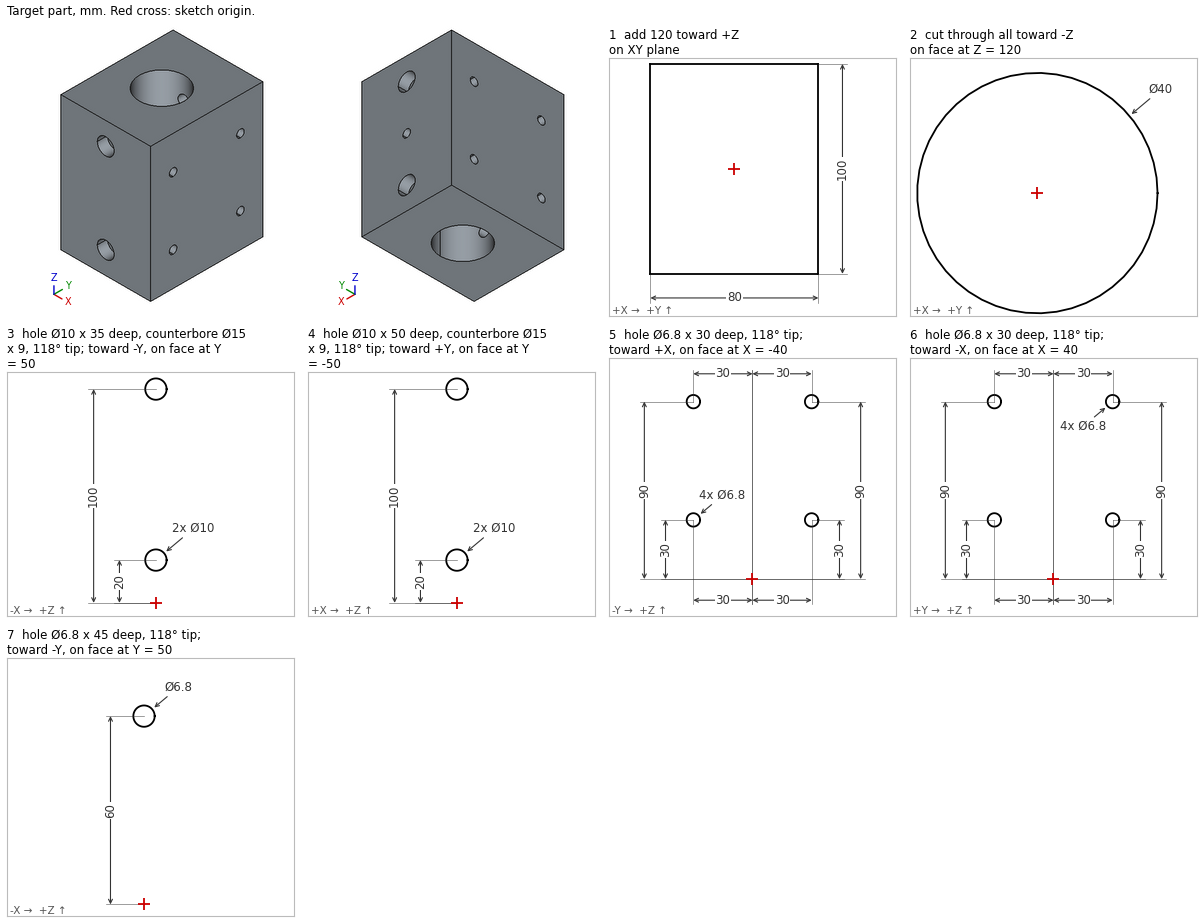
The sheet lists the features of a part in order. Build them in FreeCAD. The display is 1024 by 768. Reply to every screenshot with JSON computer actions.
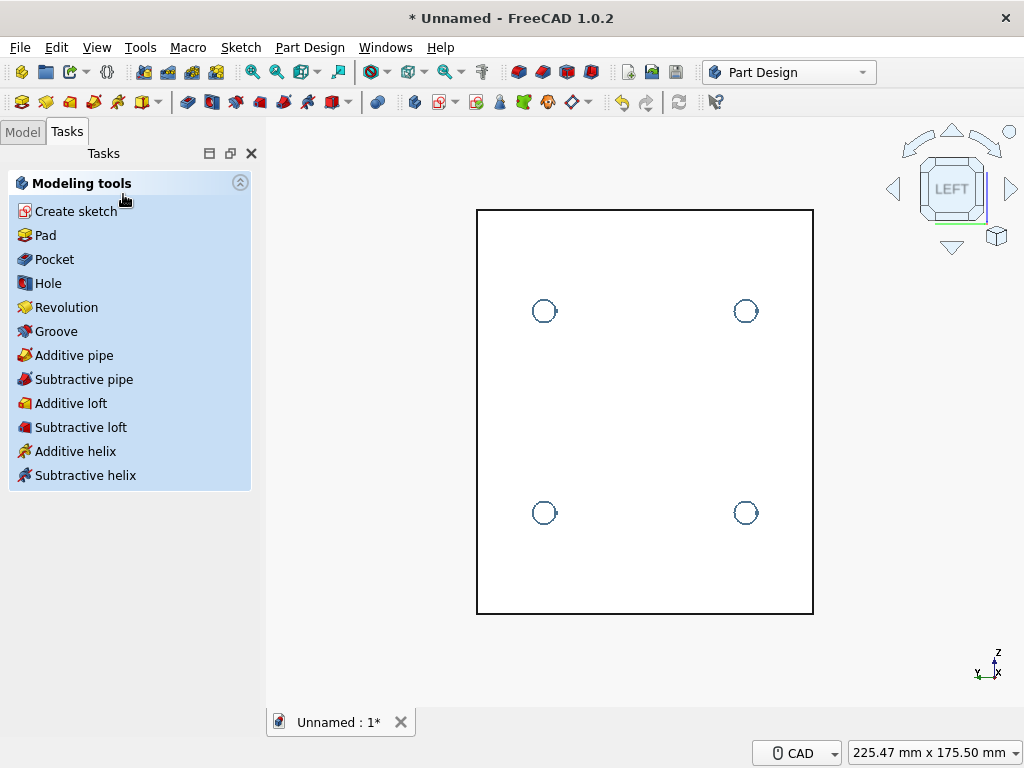
{"action": "left_click", "coordinate": [212, 102]}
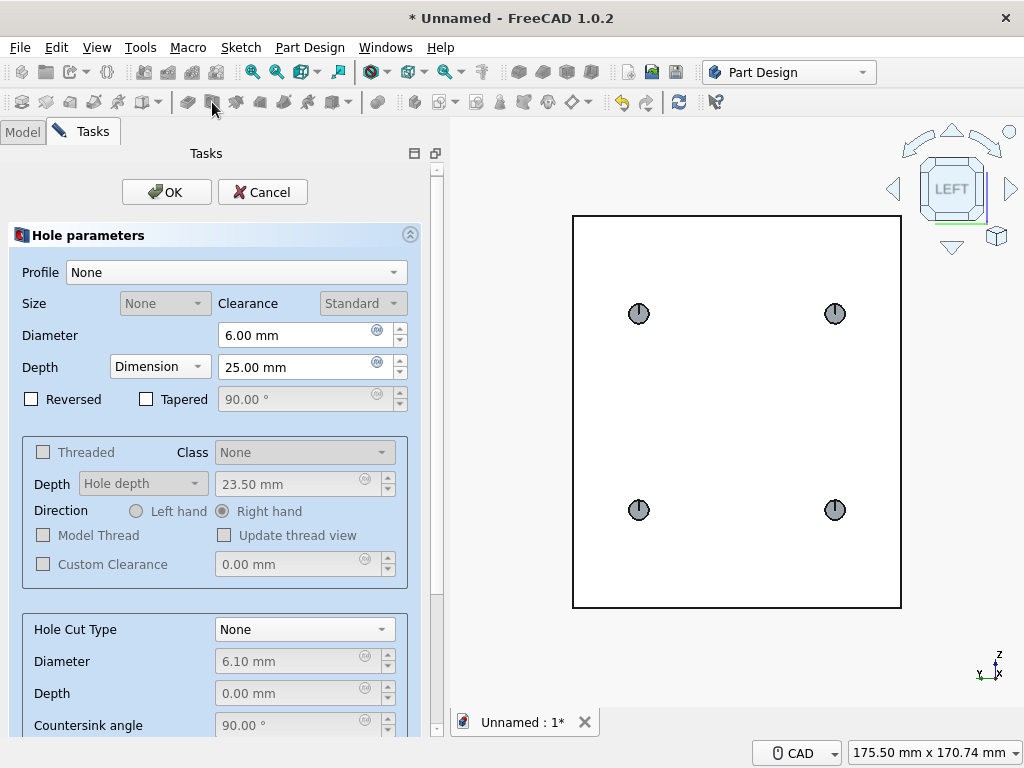
{"action": "triple_click", "coordinate": [305, 335]}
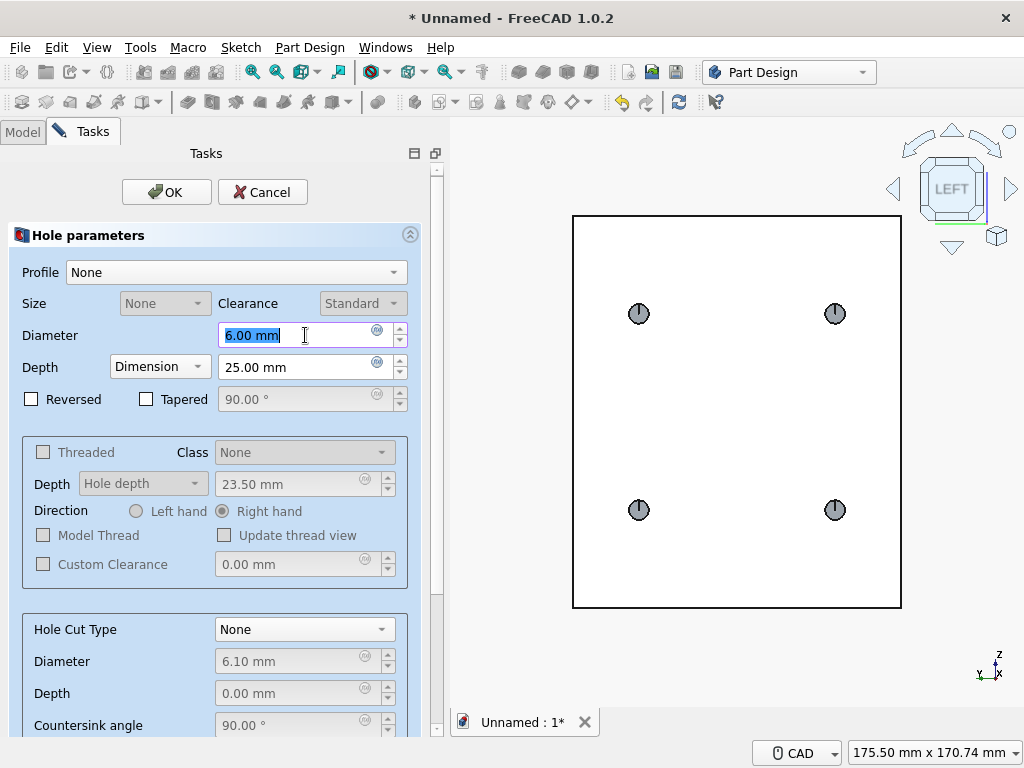
{"action": "type", "text": "6.8"}
{"action": "key", "text": "Tab"}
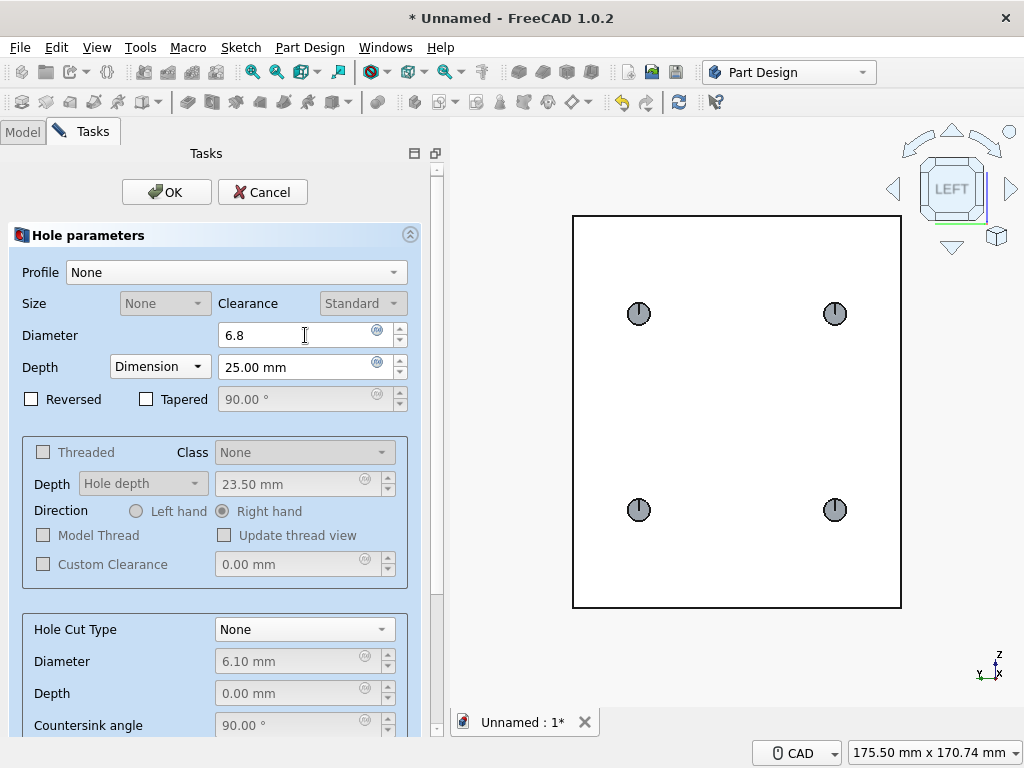
{"action": "triple_click", "coordinate": [305, 367]}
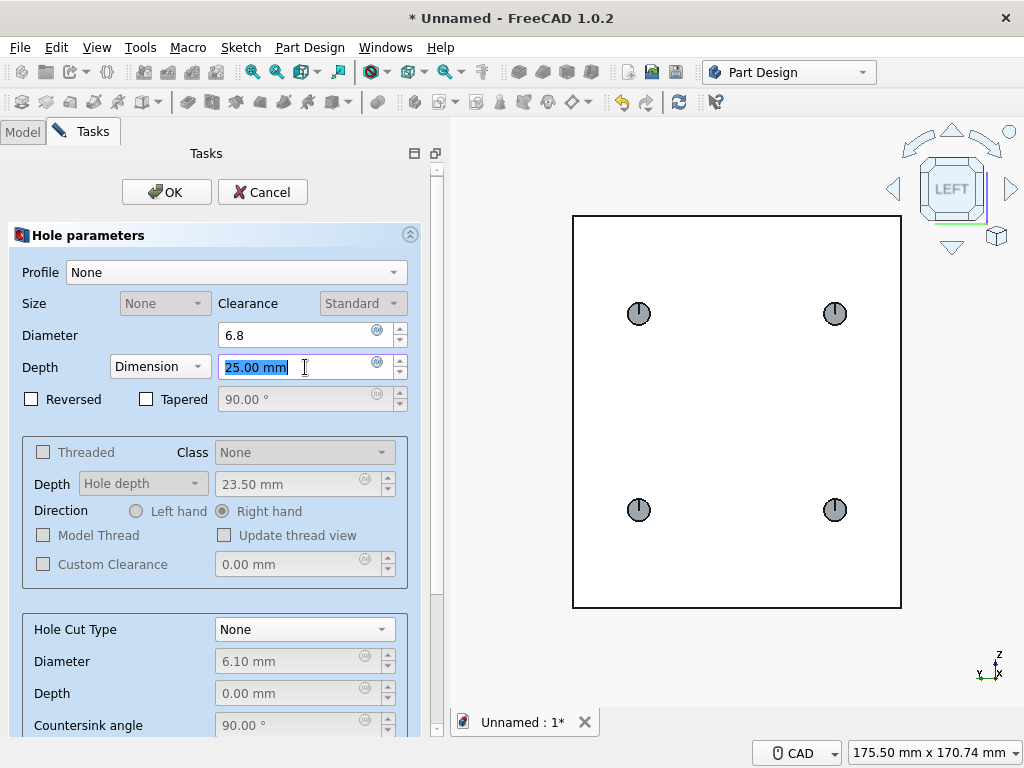
{"action": "type", "text": "30"}
{"action": "key", "text": "Tab"}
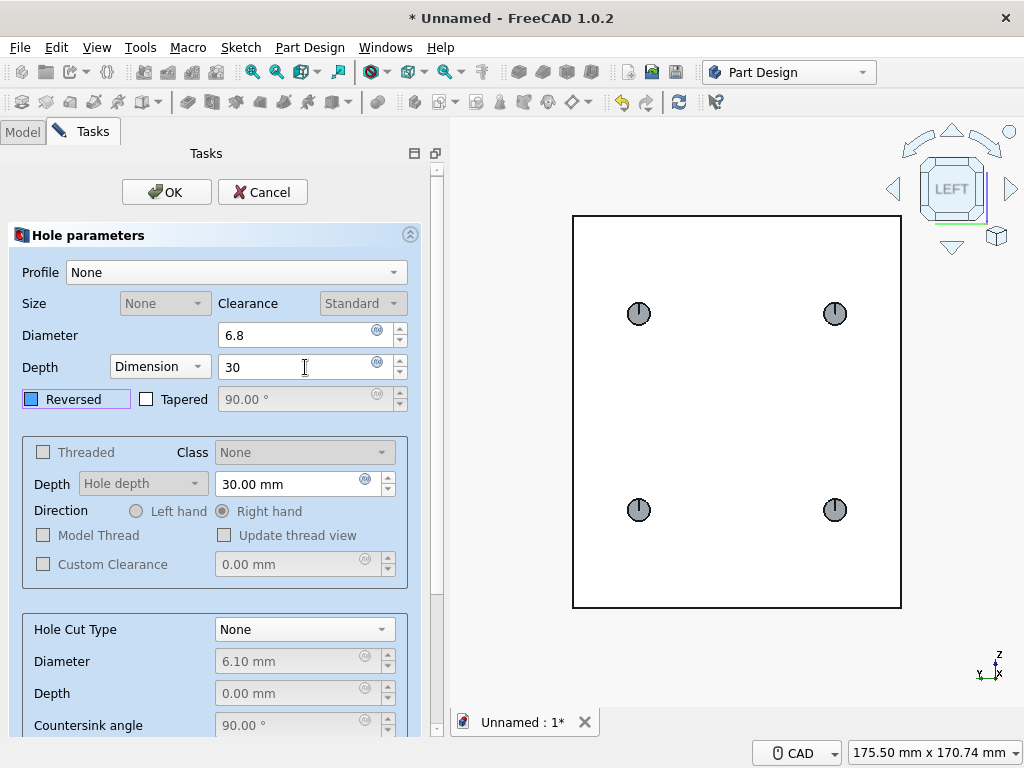
{"action": "left_click", "coordinate": [167, 192]}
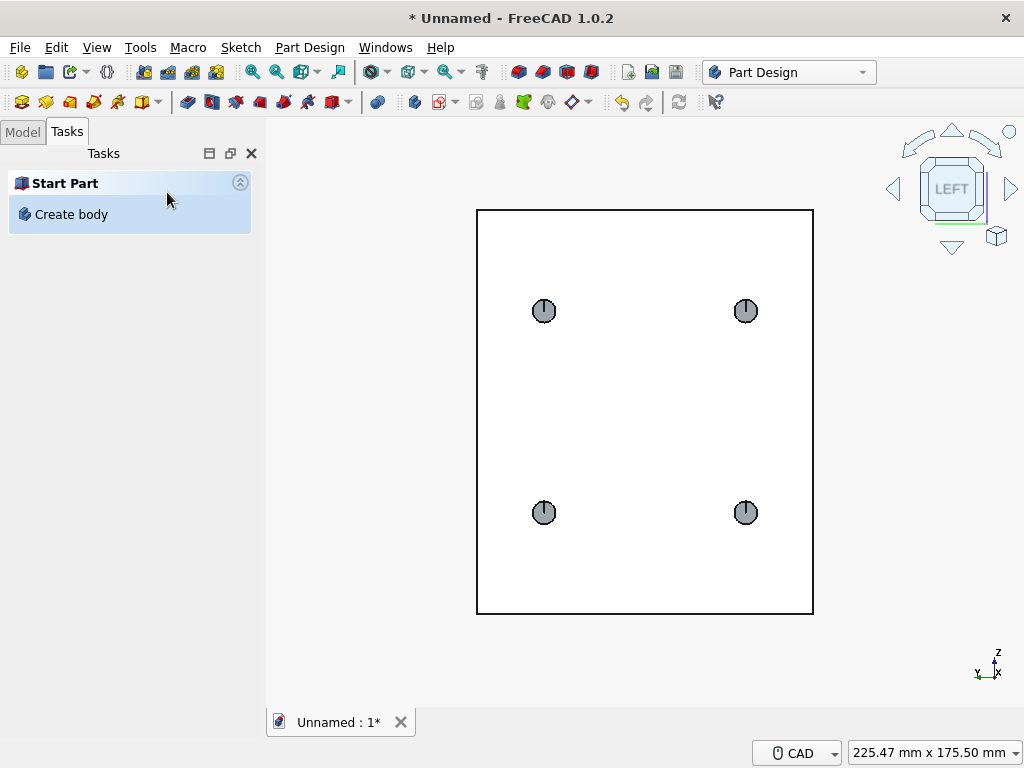
{"action": "key", "text": "0"}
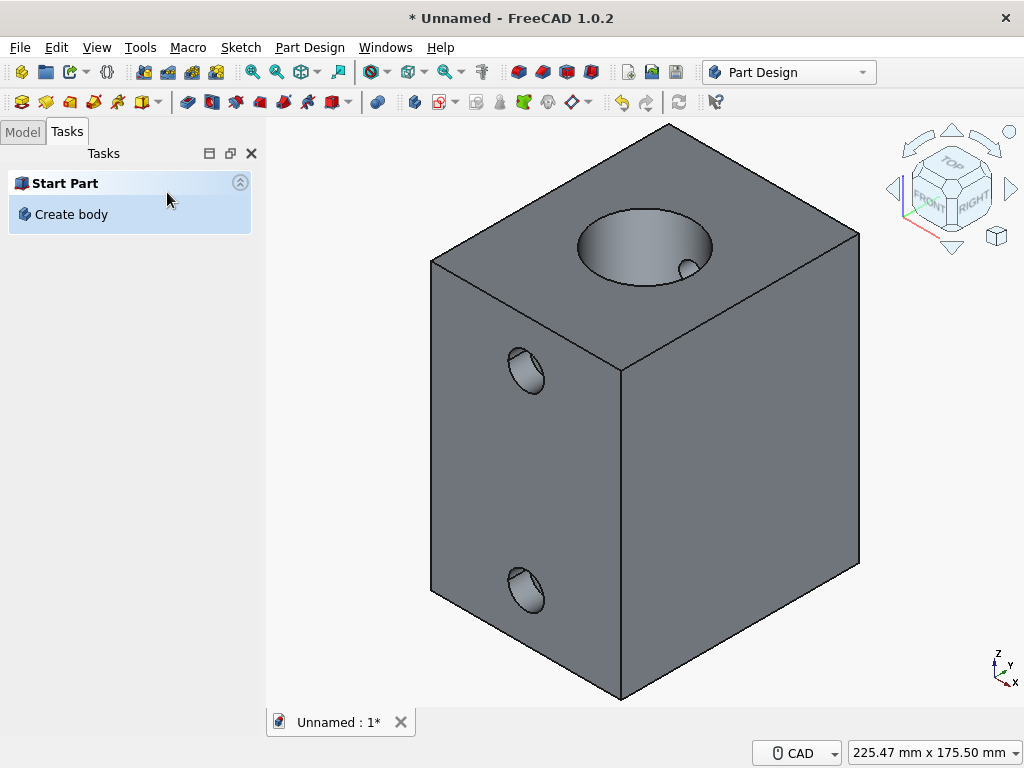
{"action": "left_click", "coordinate": [740, 466]}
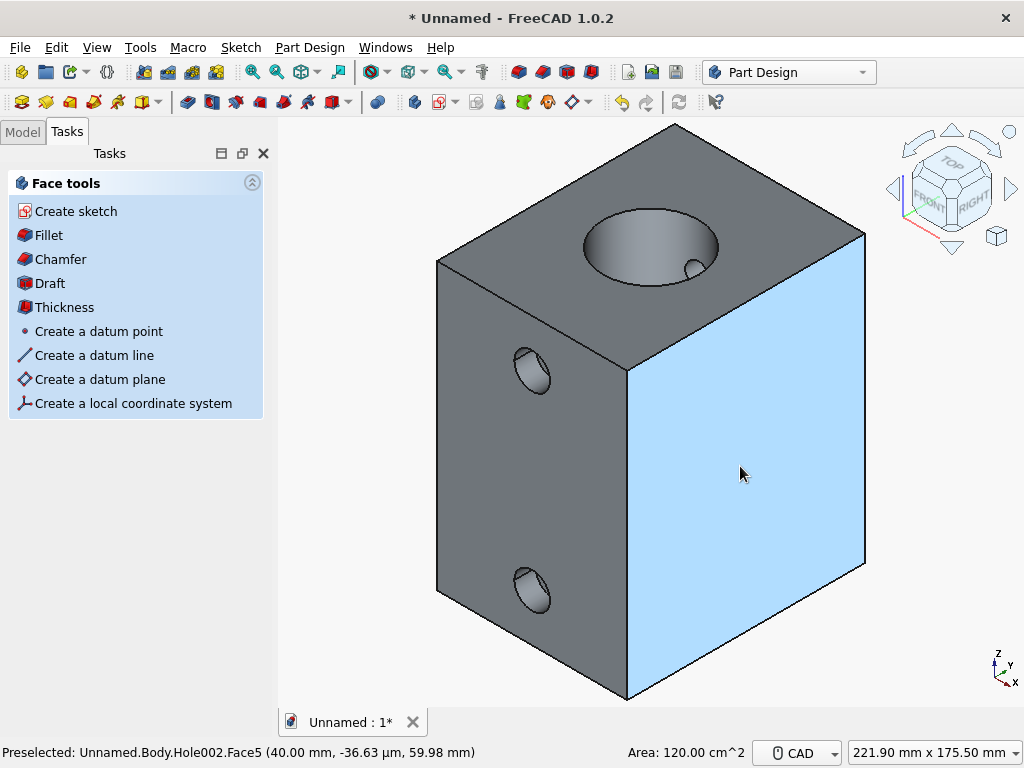
{"action": "left_click", "coordinate": [440, 102]}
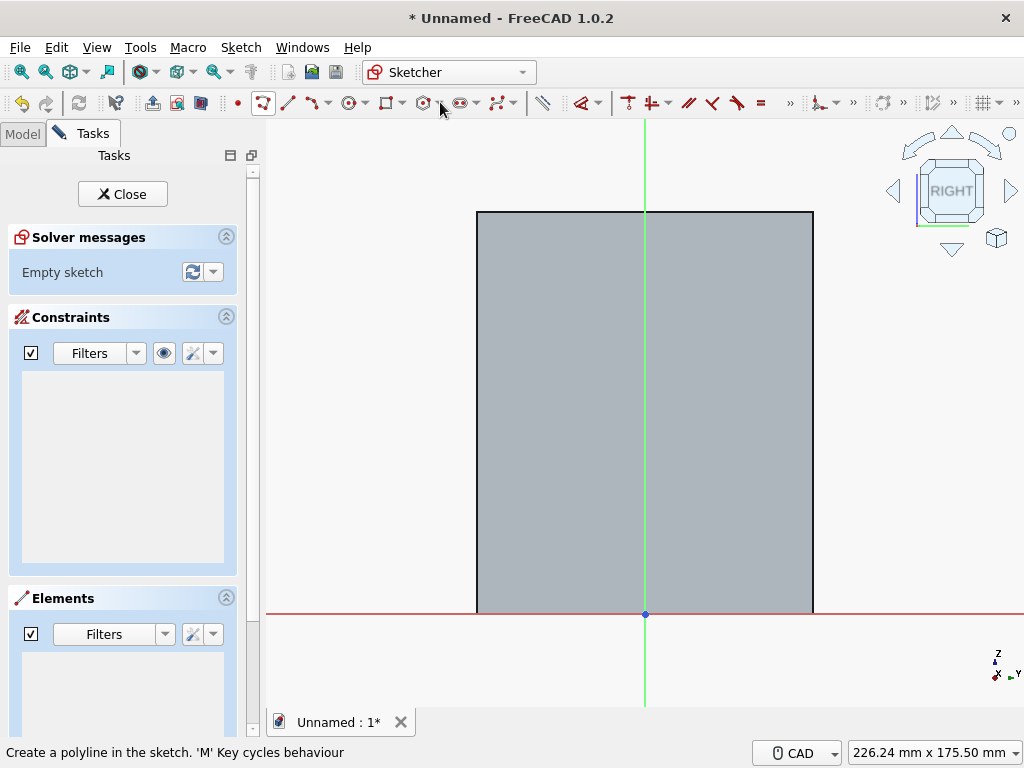
{"action": "left_click", "coordinate": [350, 104]}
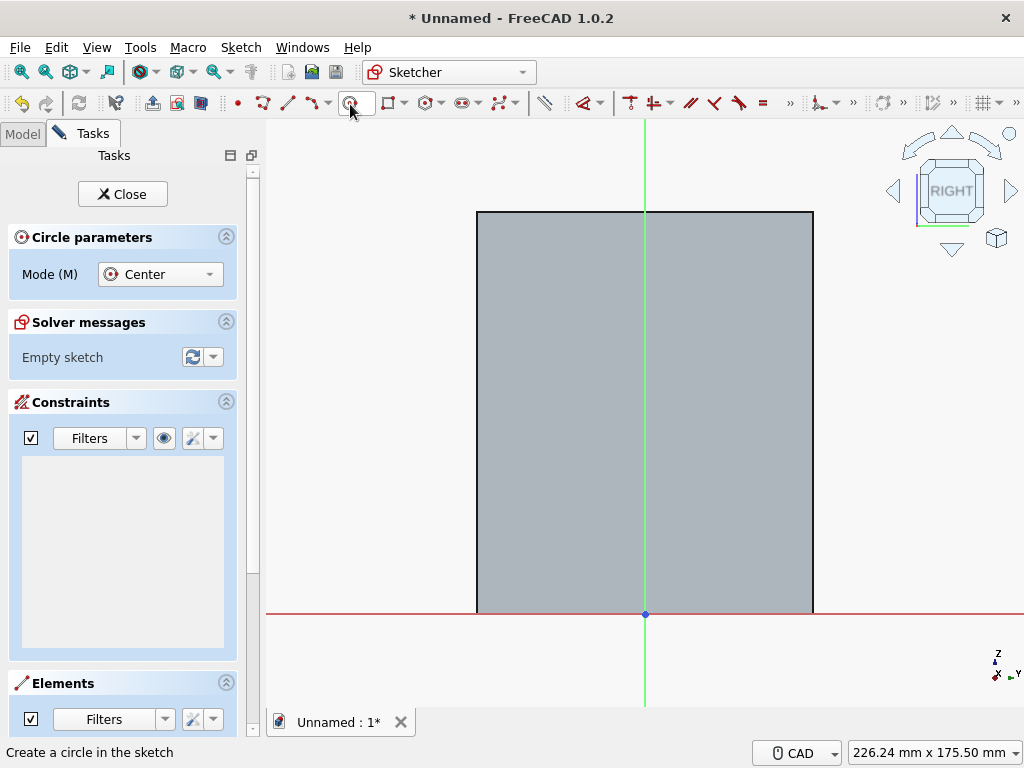
{"action": "scroll", "coordinate": [746, 312], "scroll_direction": "up", "scroll_amount": 4}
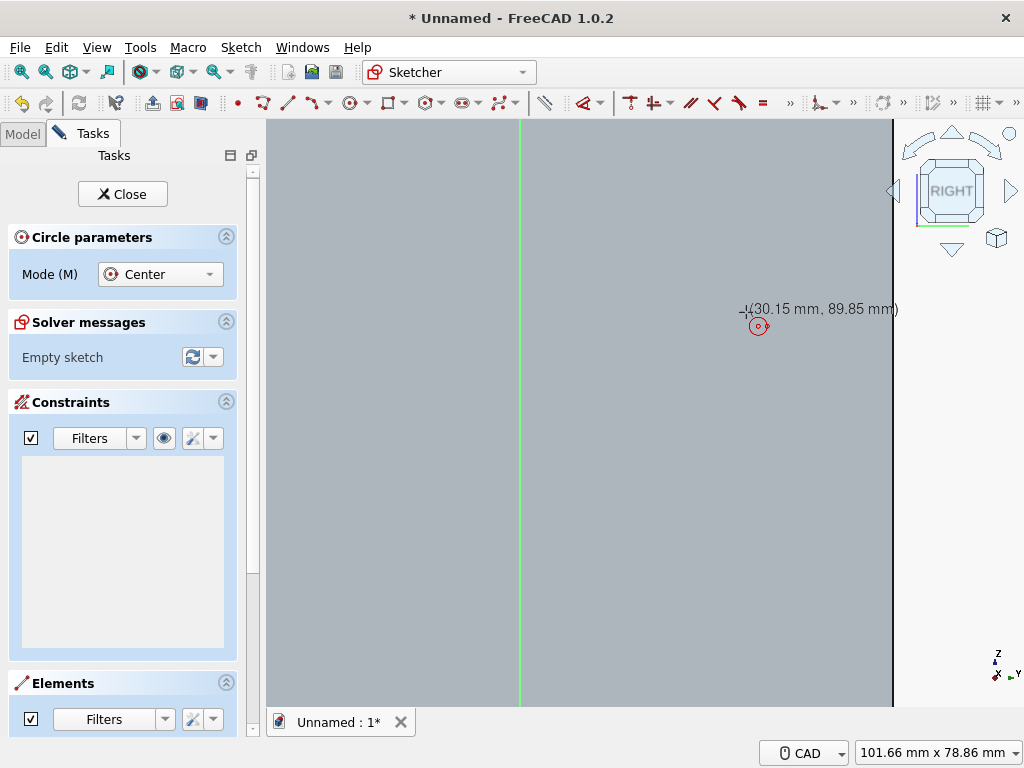
{"action": "left_click", "coordinate": [744, 313]}
{"action": "mouse_move", "coordinate": [762, 295]}